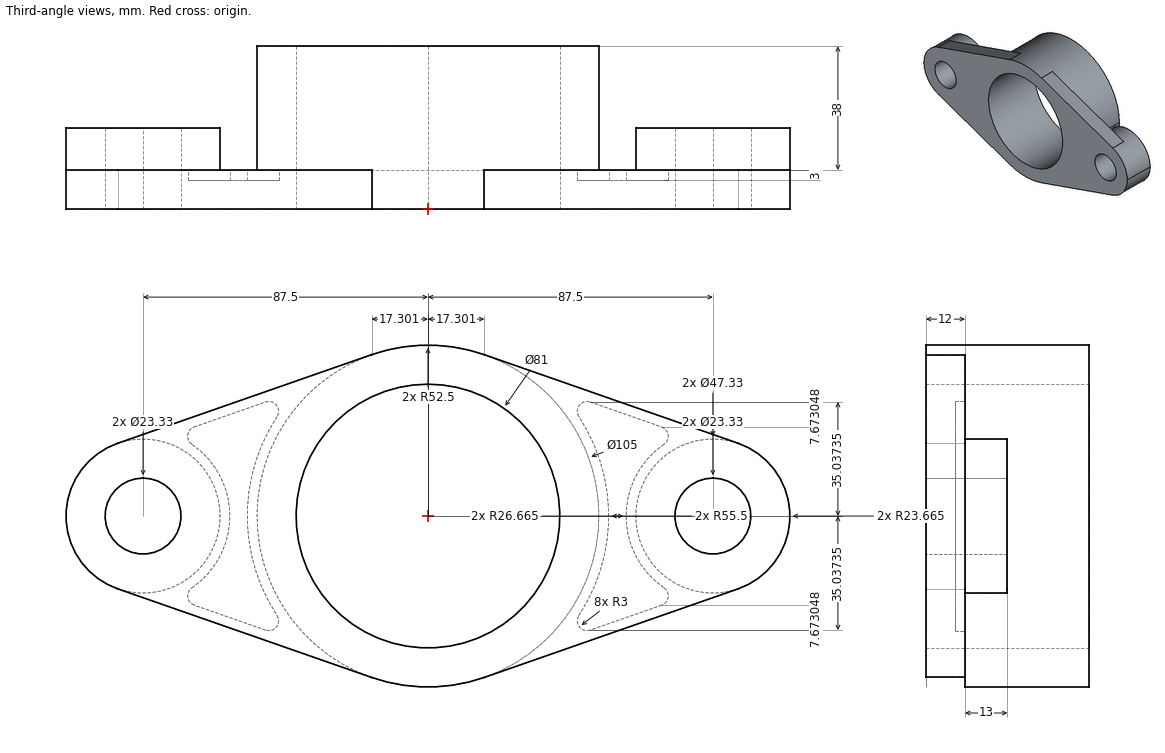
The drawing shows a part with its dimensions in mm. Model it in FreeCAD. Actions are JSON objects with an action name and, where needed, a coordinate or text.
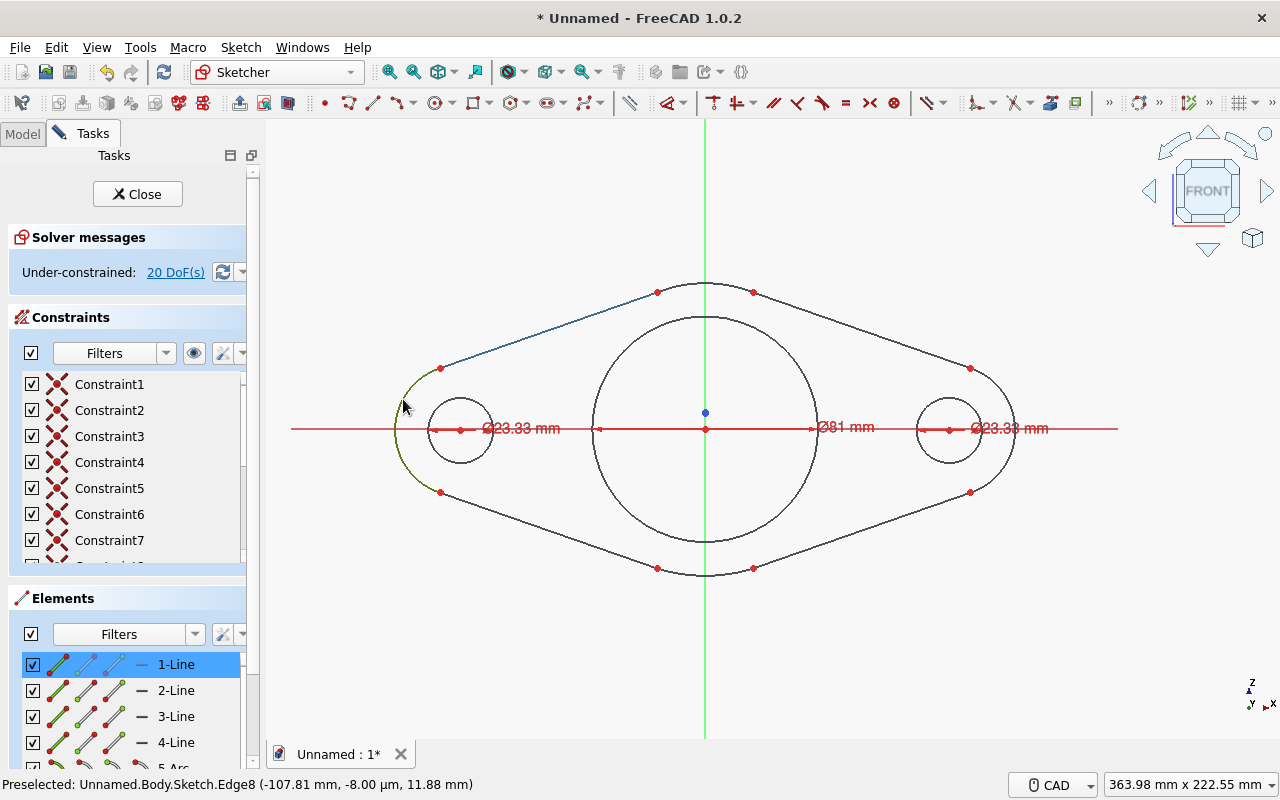
{"action": "left_click", "coordinate": [822, 104]}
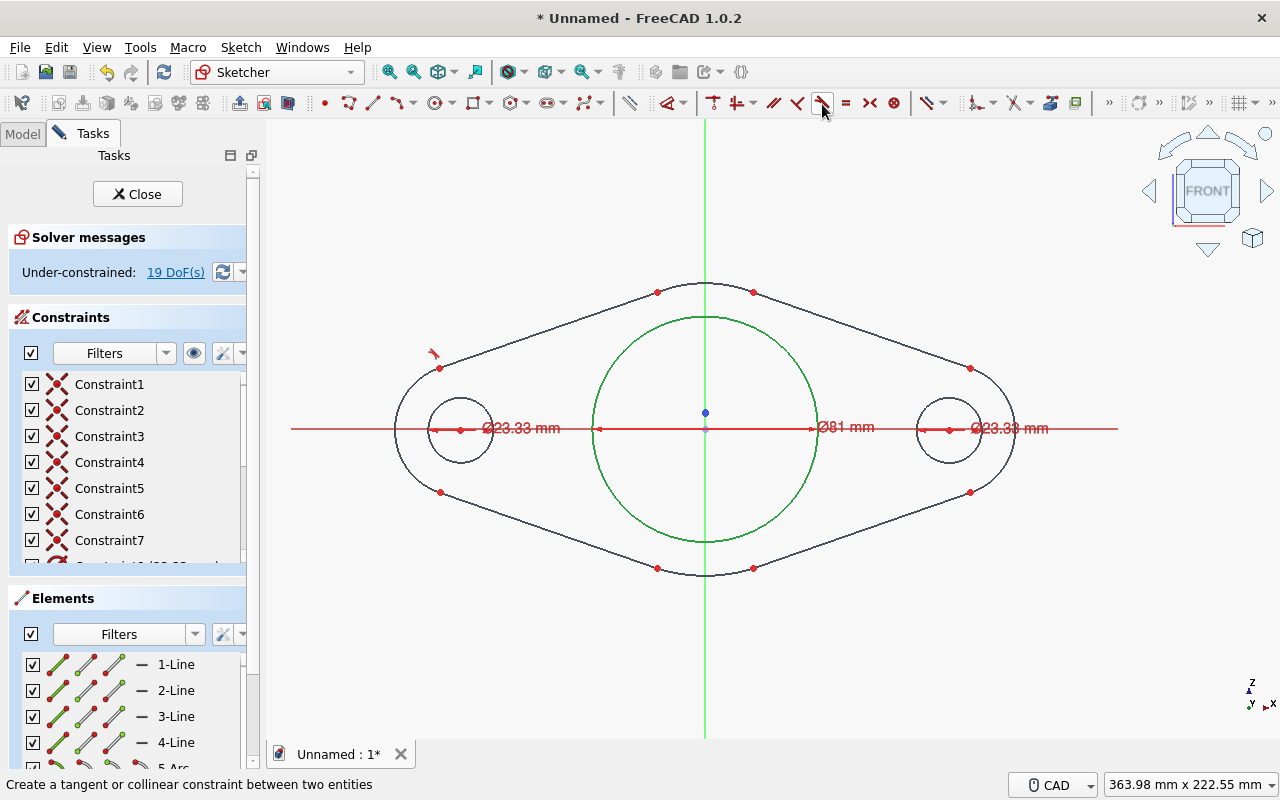
{"action": "left_click", "coordinate": [818, 315]}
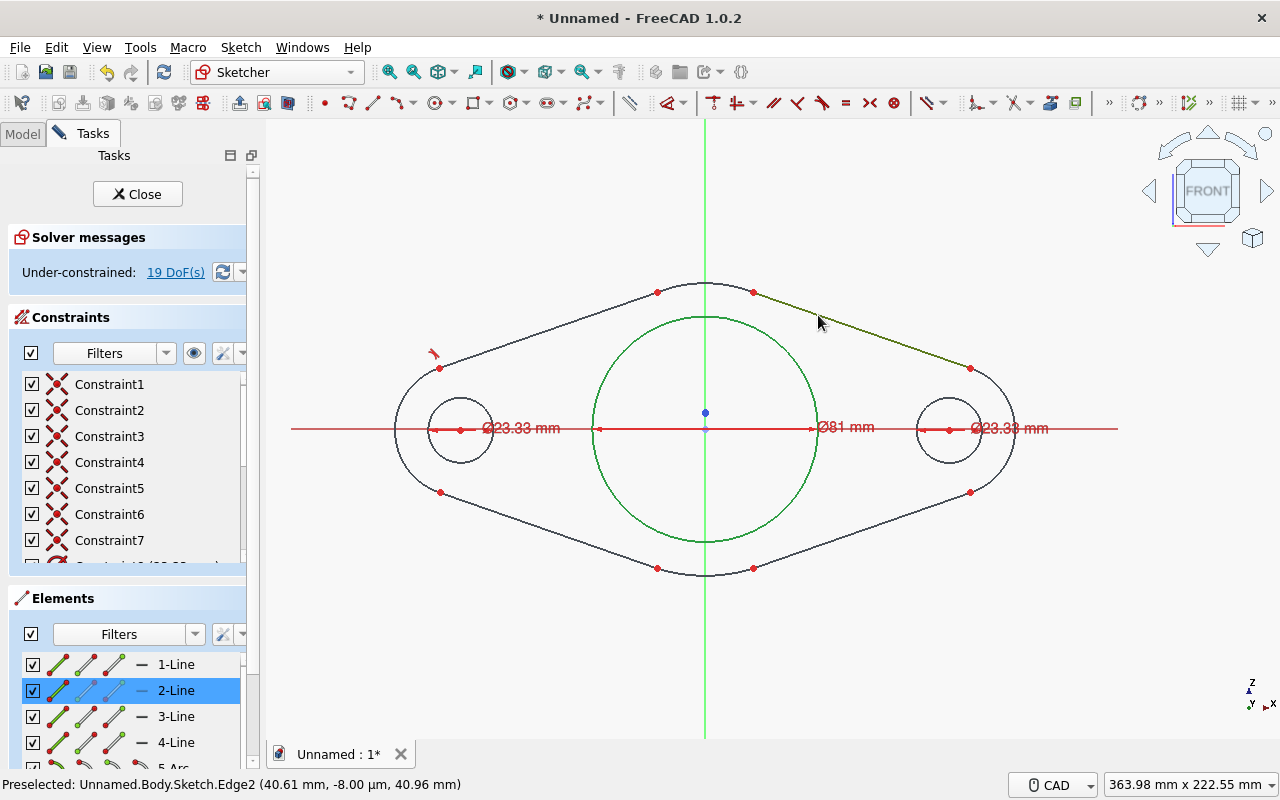
{"action": "left_click", "coordinate": [1007, 462]}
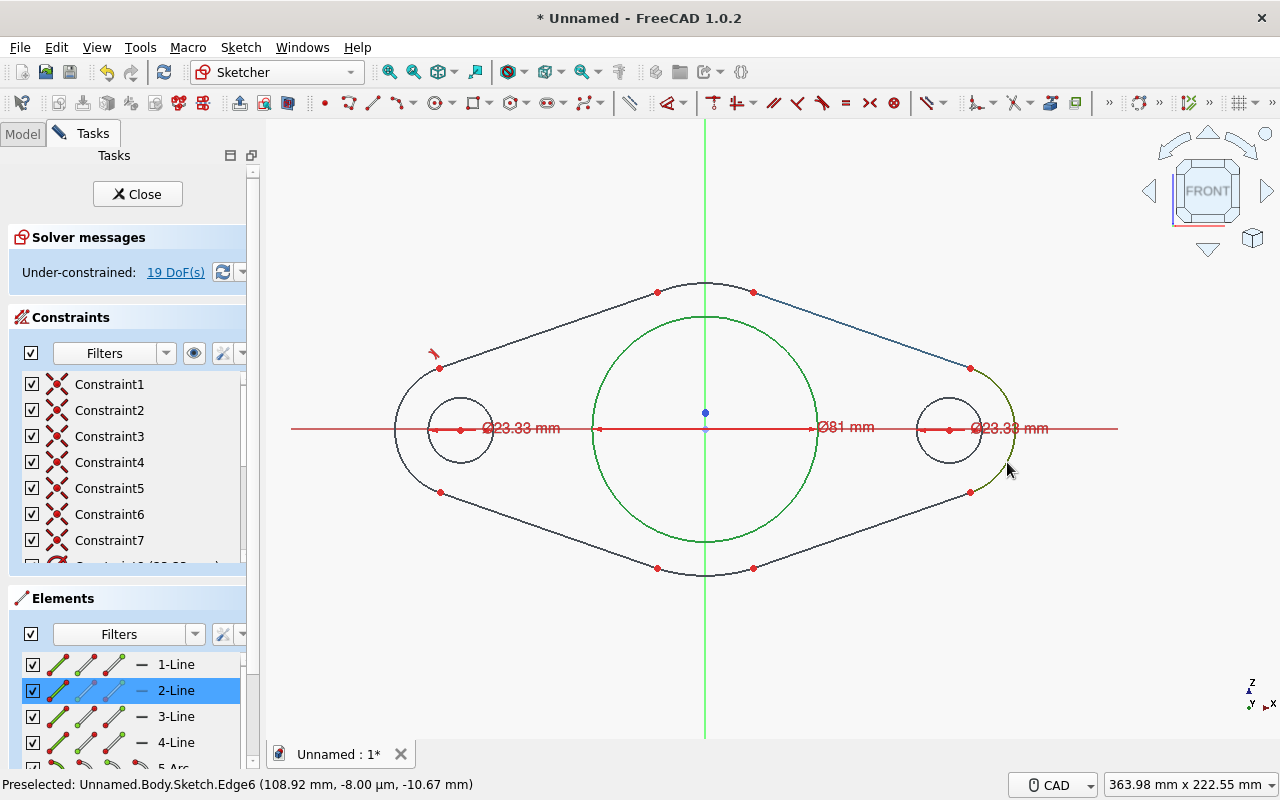
{"action": "left_click", "coordinate": [822, 104]}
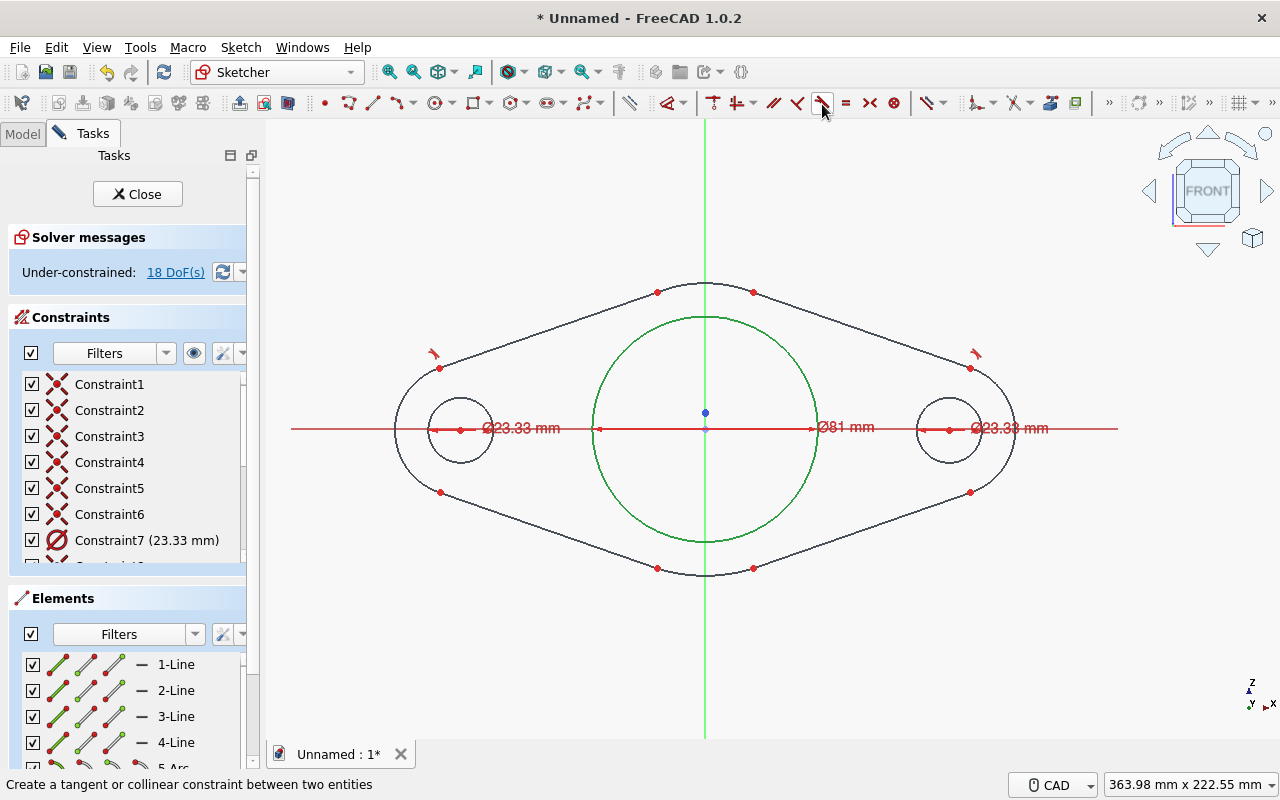
{"action": "left_click", "coordinate": [905, 516]}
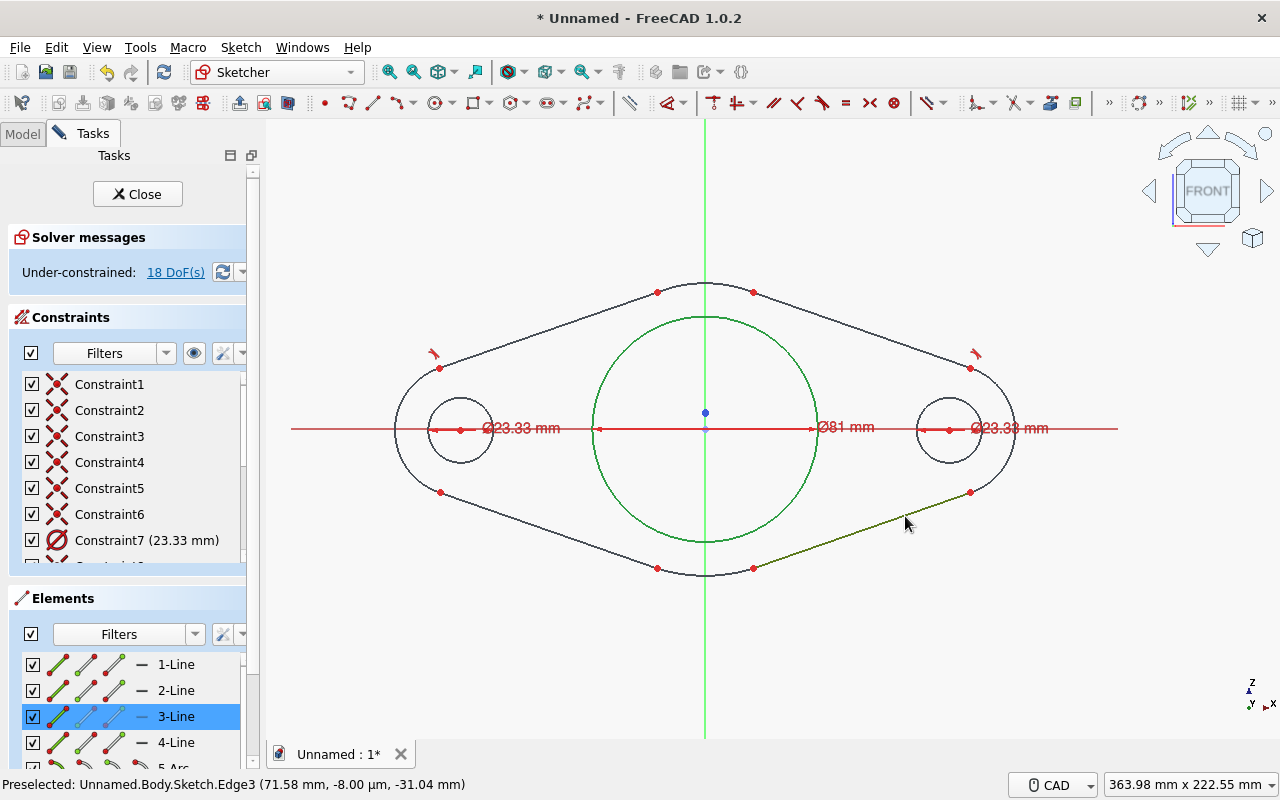
{"action": "left_click", "coordinate": [1007, 462]}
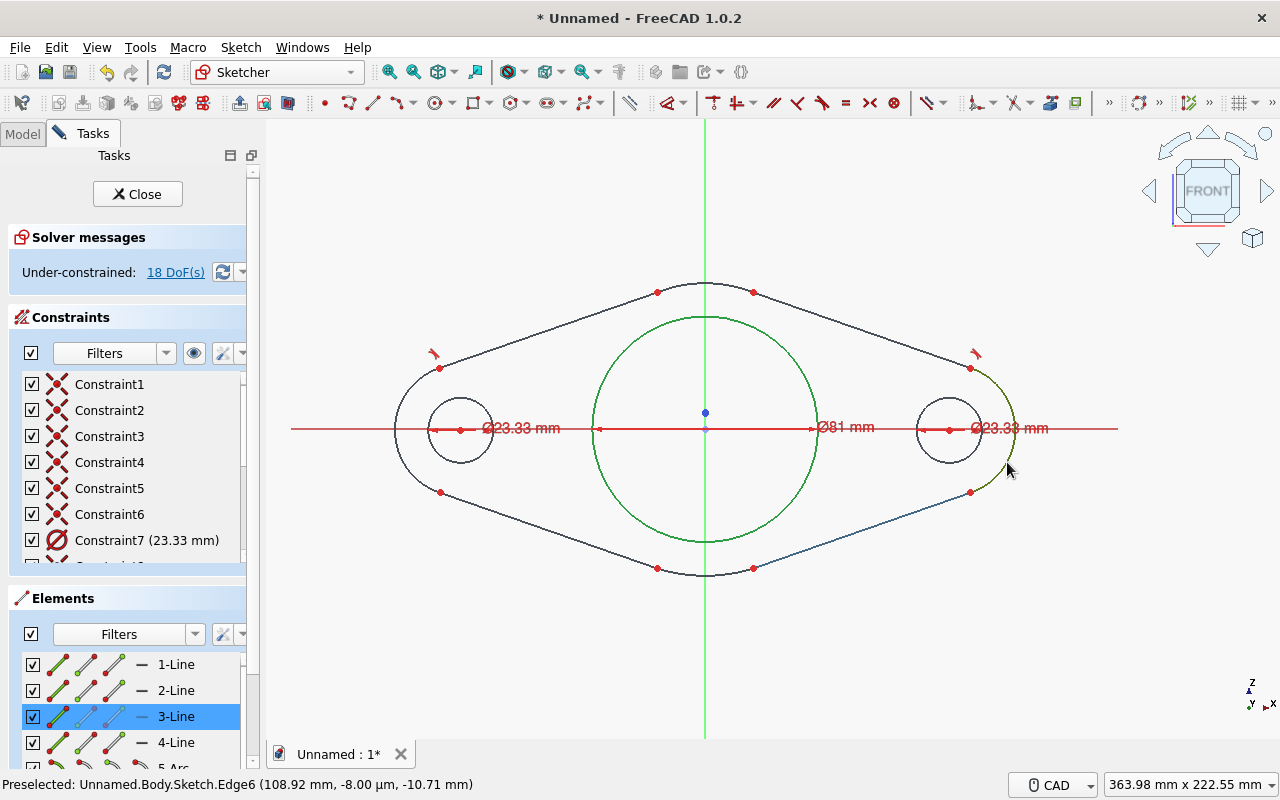
{"action": "left_click", "coordinate": [822, 104]}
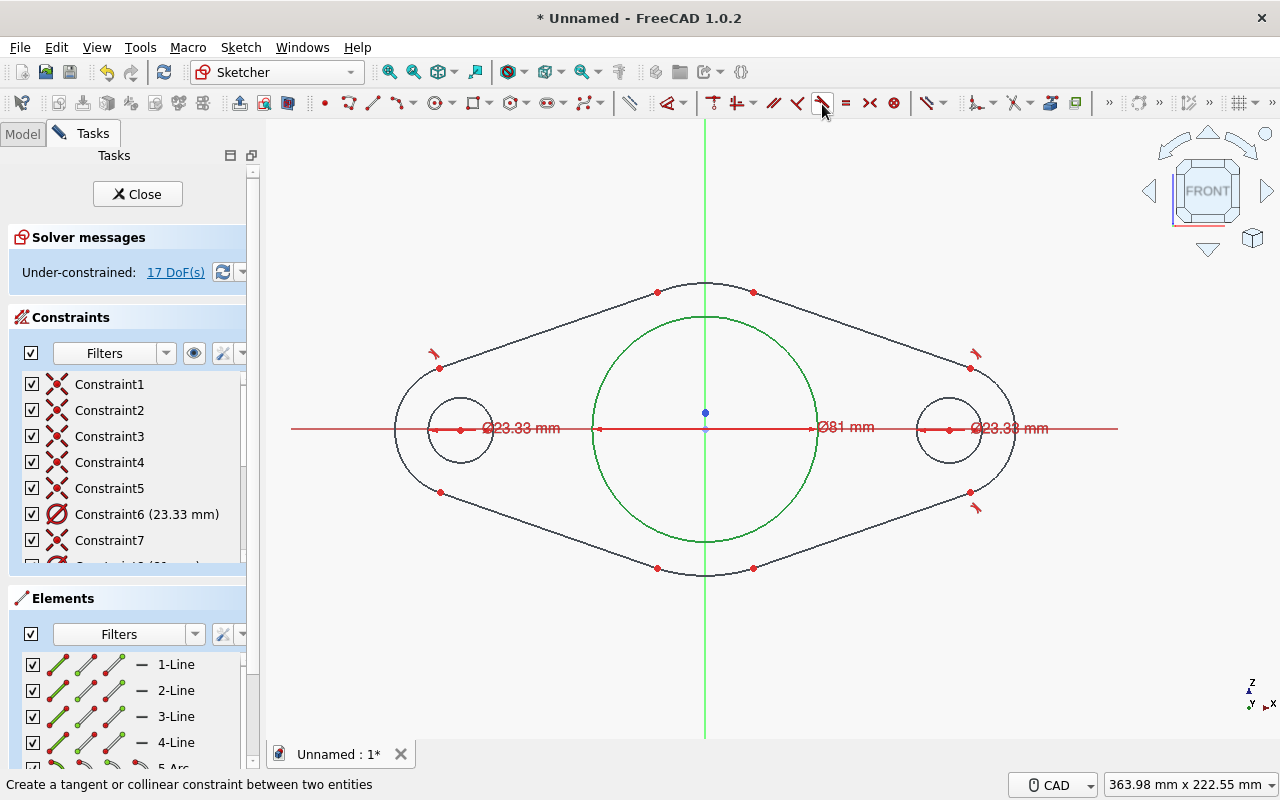
{"action": "left_click", "coordinate": [592, 546]}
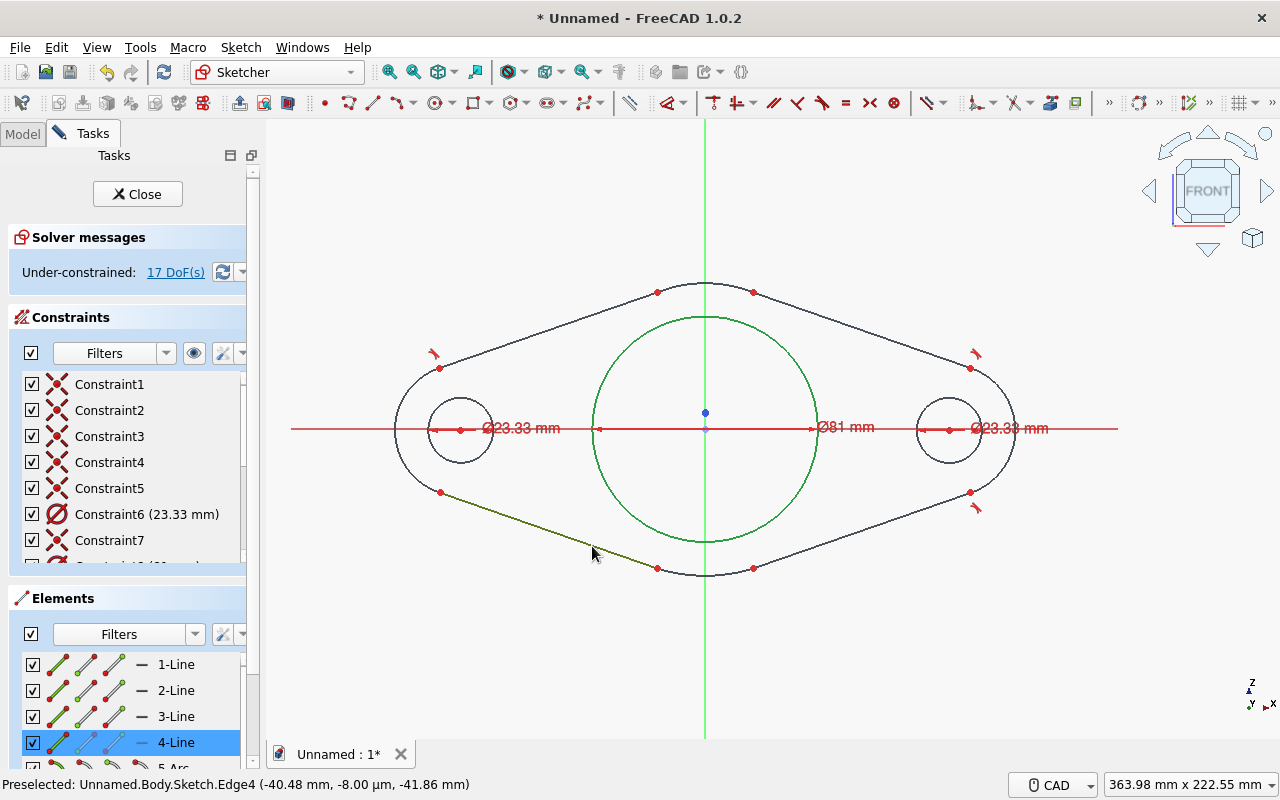
{"action": "left_click", "coordinate": [403, 399]}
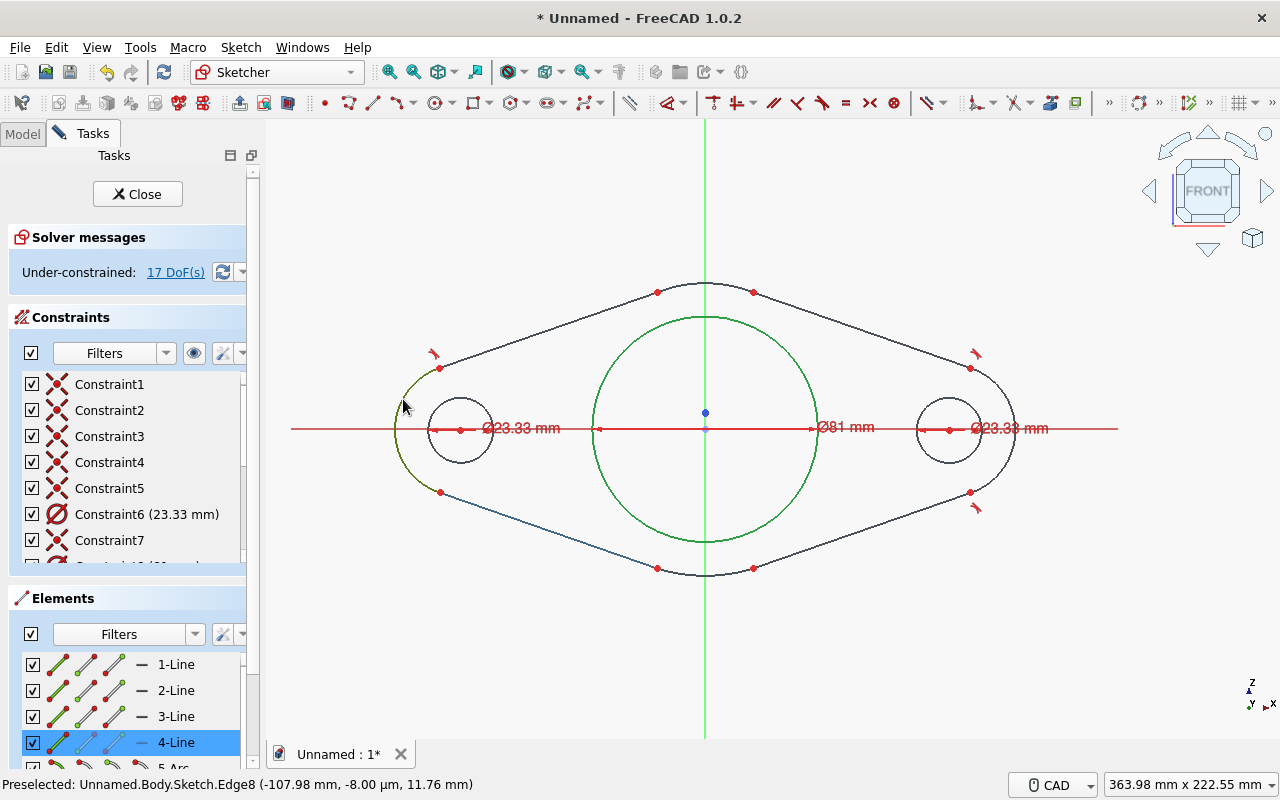
{"action": "left_click", "coordinate": [822, 104]}